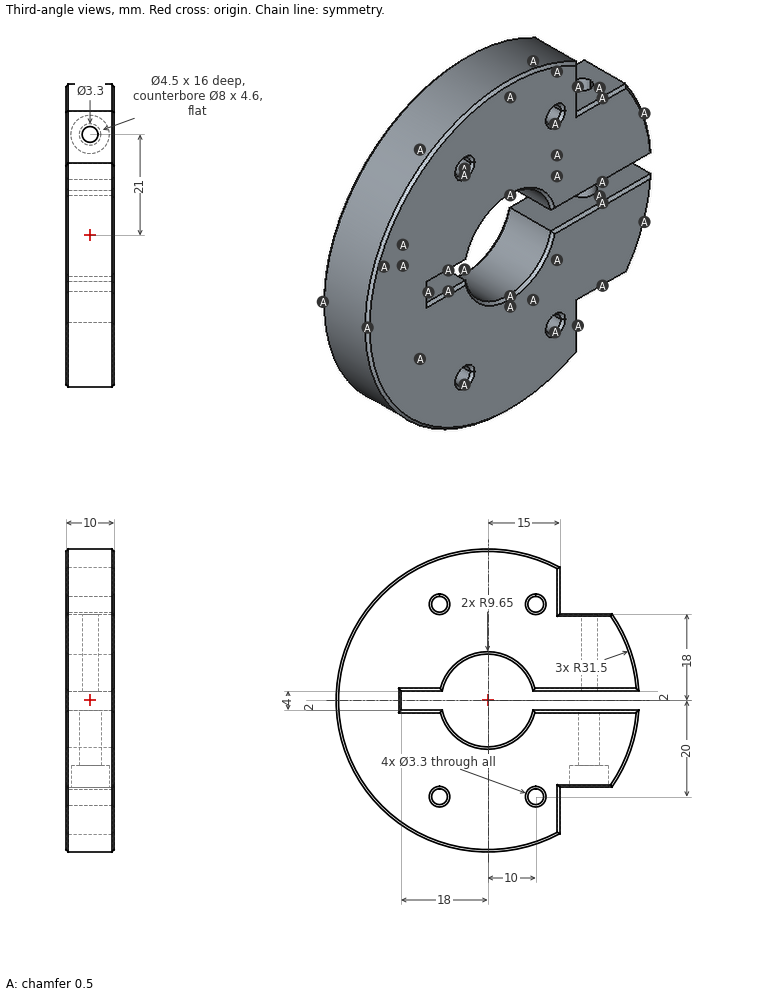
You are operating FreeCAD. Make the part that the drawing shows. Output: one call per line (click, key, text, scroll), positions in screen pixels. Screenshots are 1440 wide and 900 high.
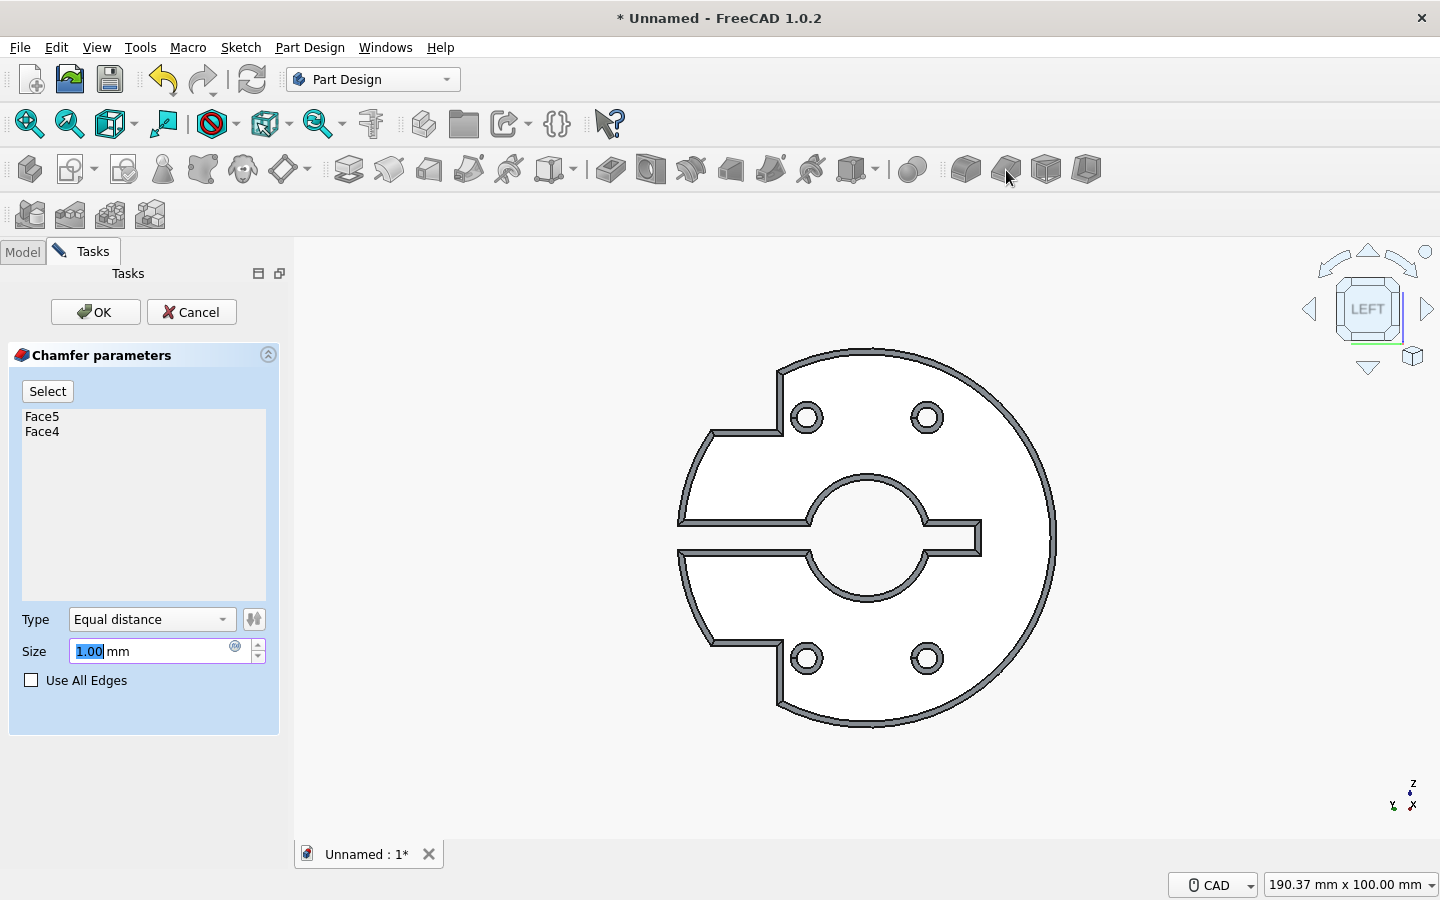
text(0.5)
key(Tab)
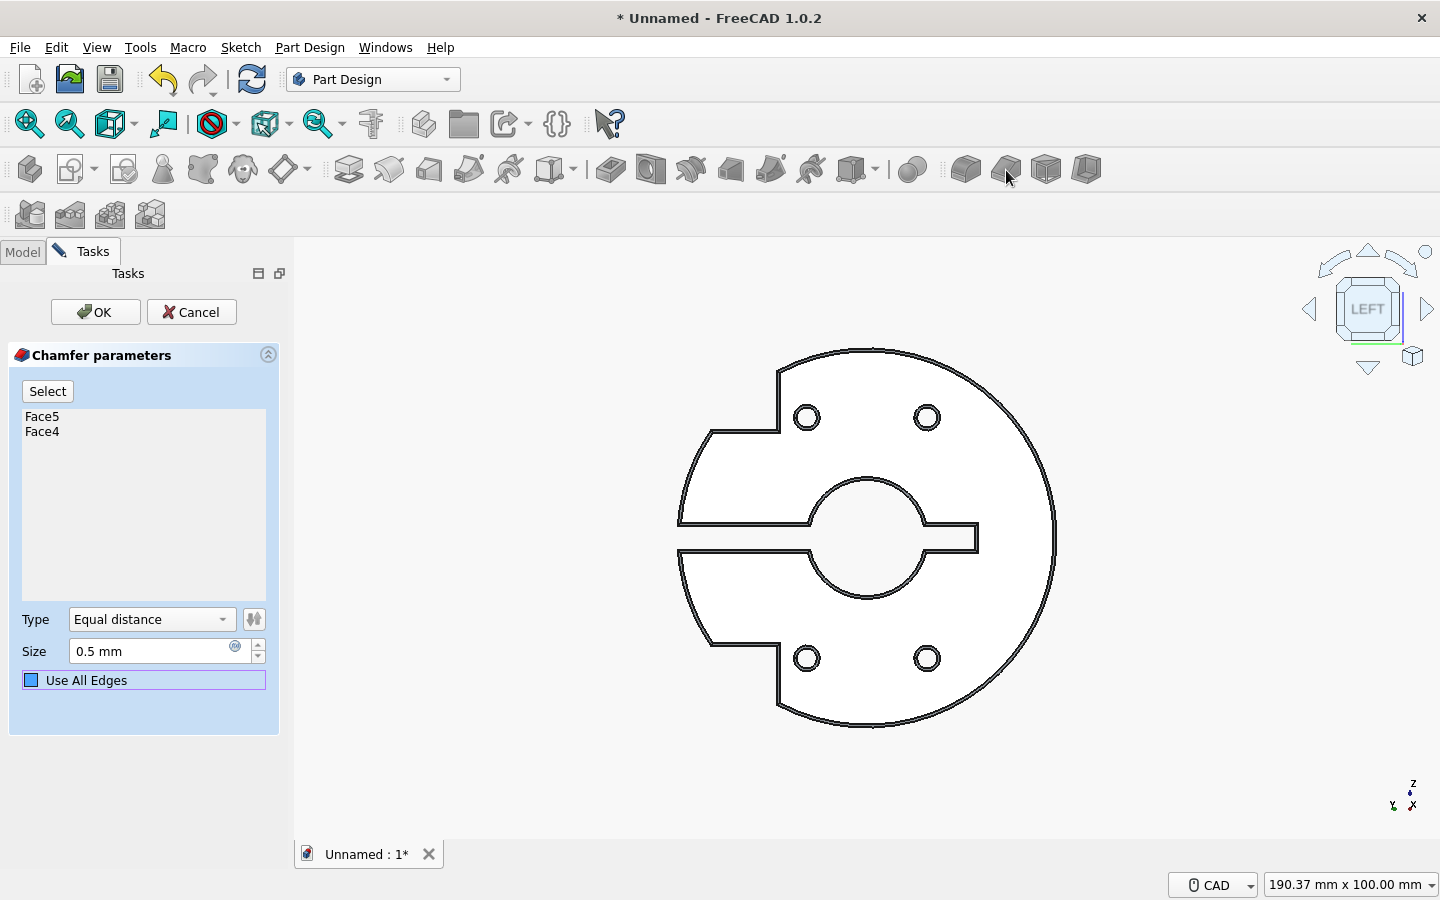
click(96, 312)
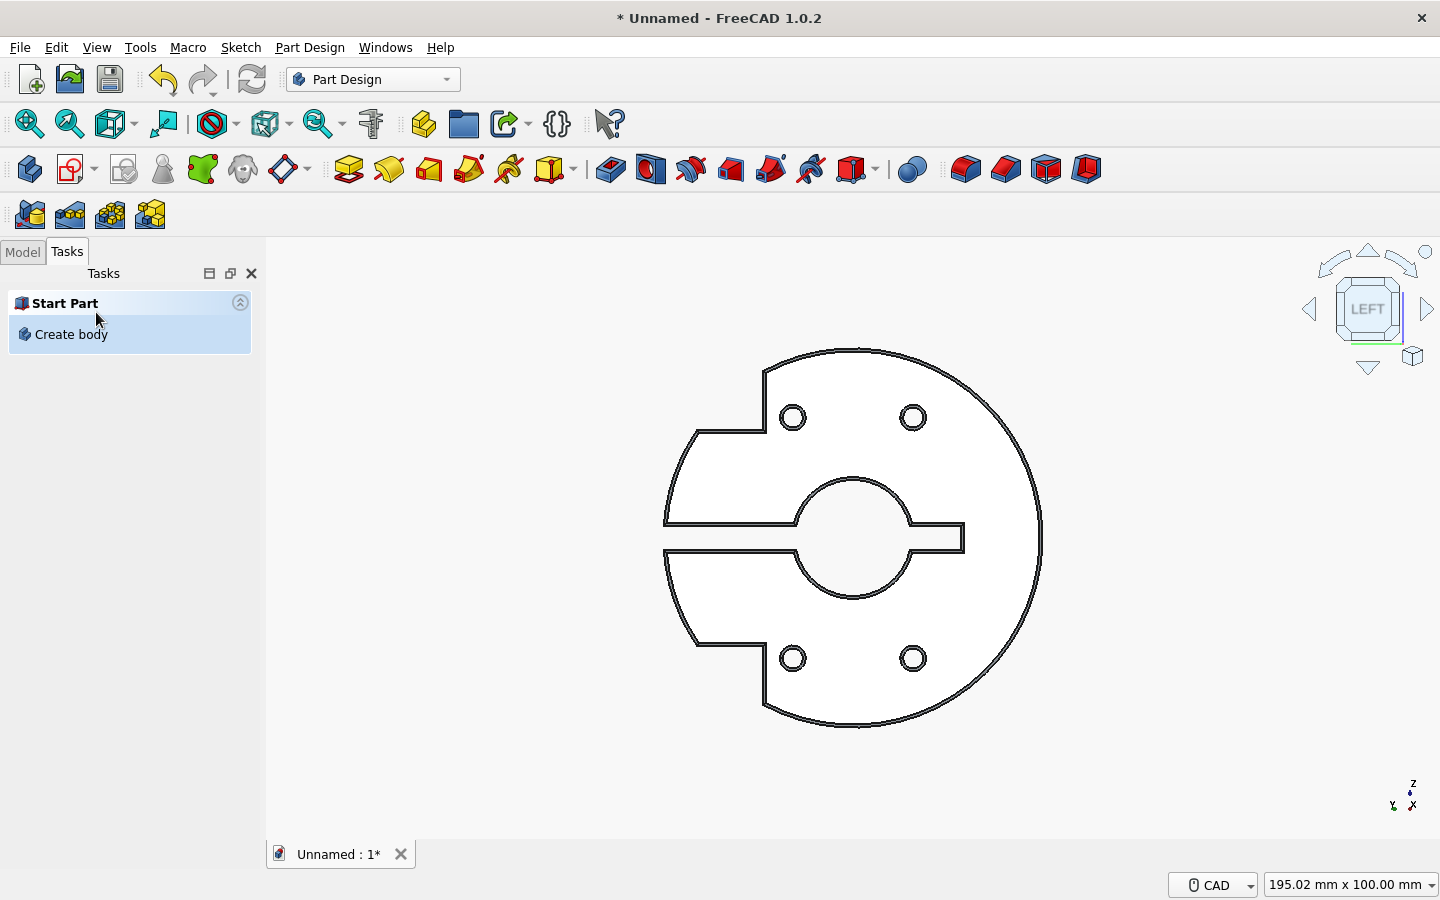
key(0)